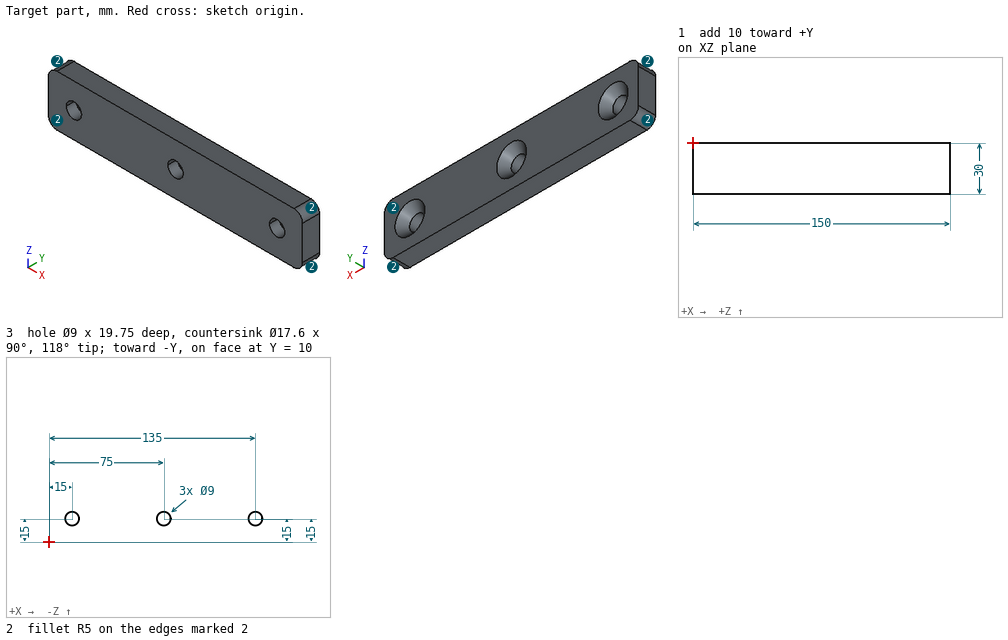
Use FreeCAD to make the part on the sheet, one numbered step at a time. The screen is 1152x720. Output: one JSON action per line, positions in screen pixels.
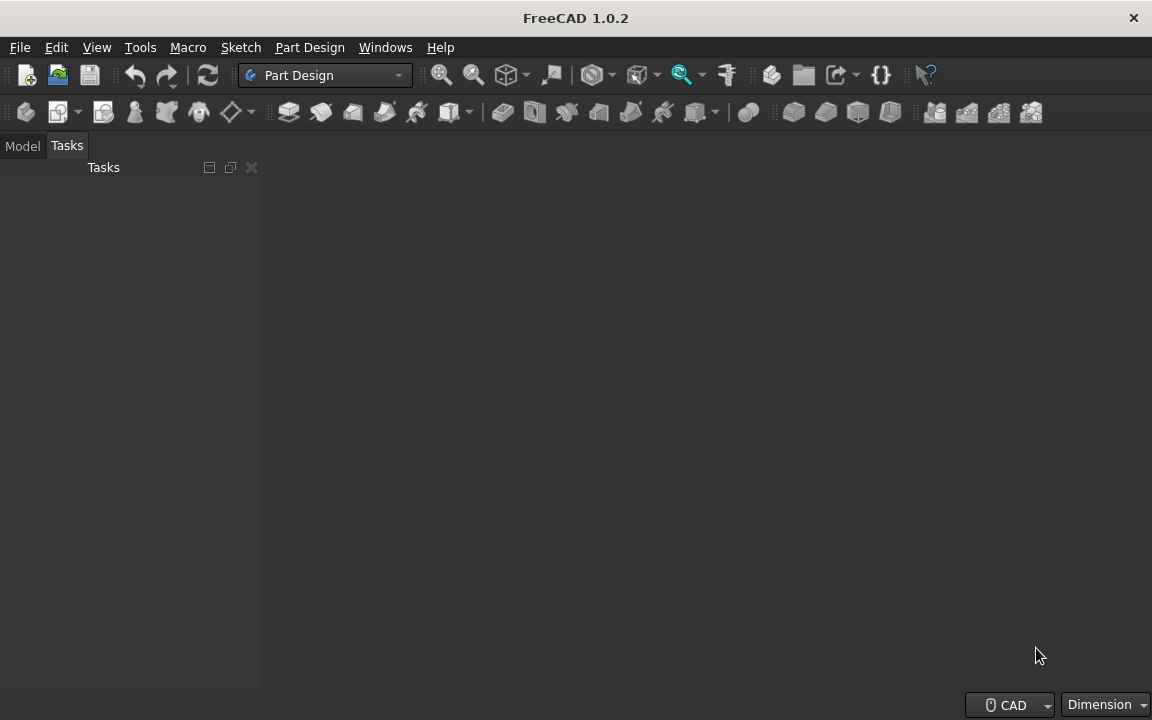
{"action": "left_click", "coordinate": [26, 76]}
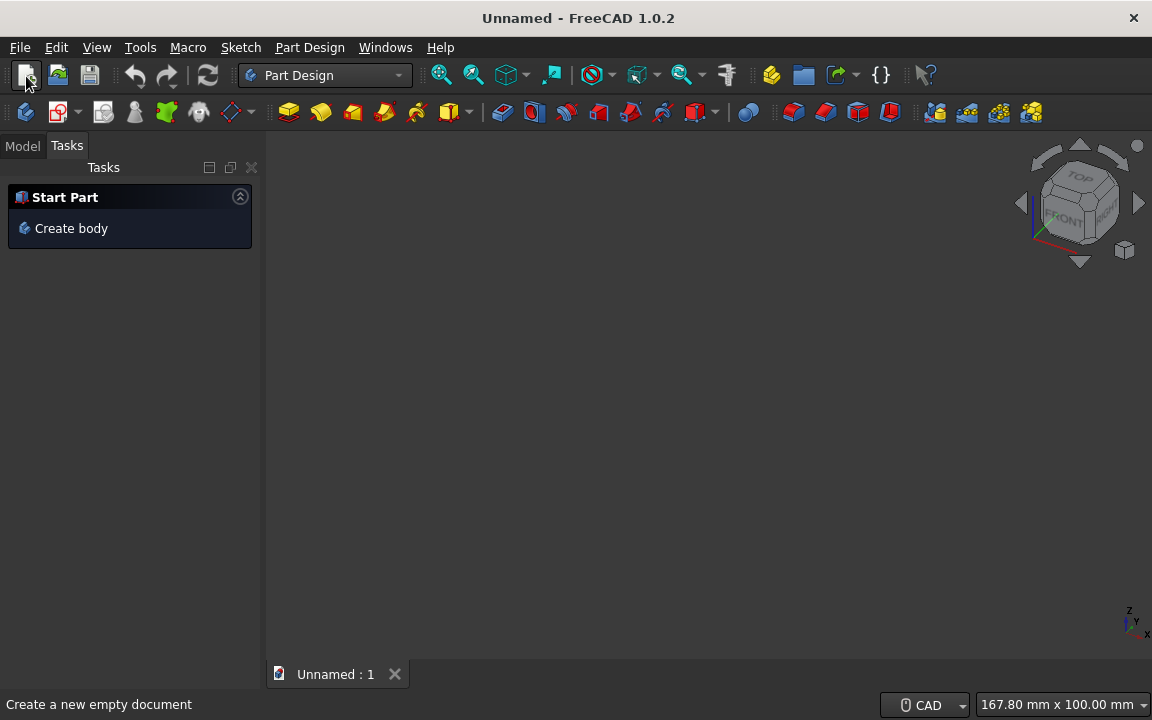
{"action": "left_click", "coordinate": [58, 112]}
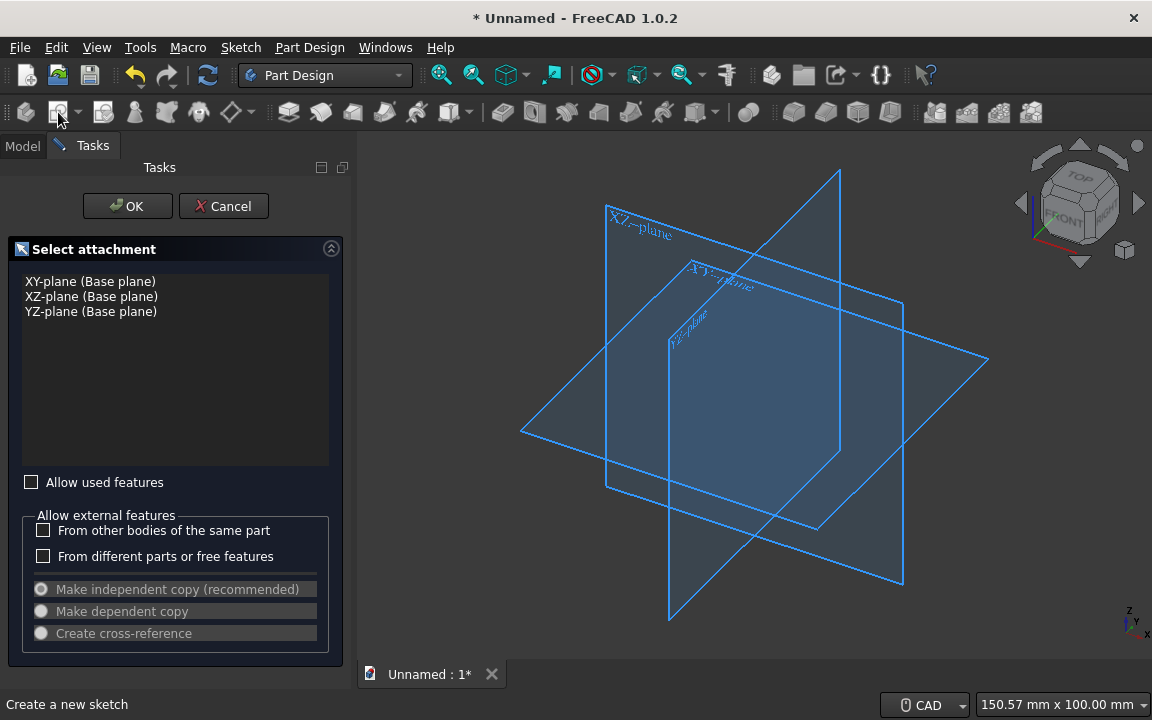
{"action": "left_click", "coordinate": [82, 296]}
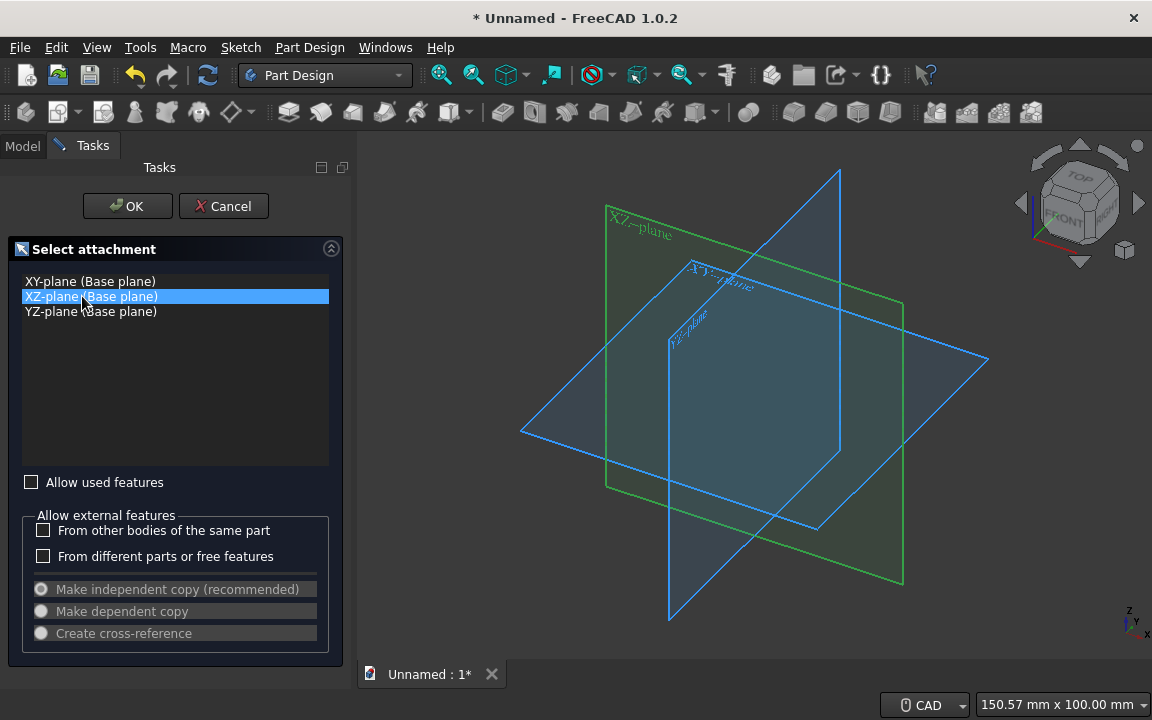
{"action": "left_click", "coordinate": [128, 206]}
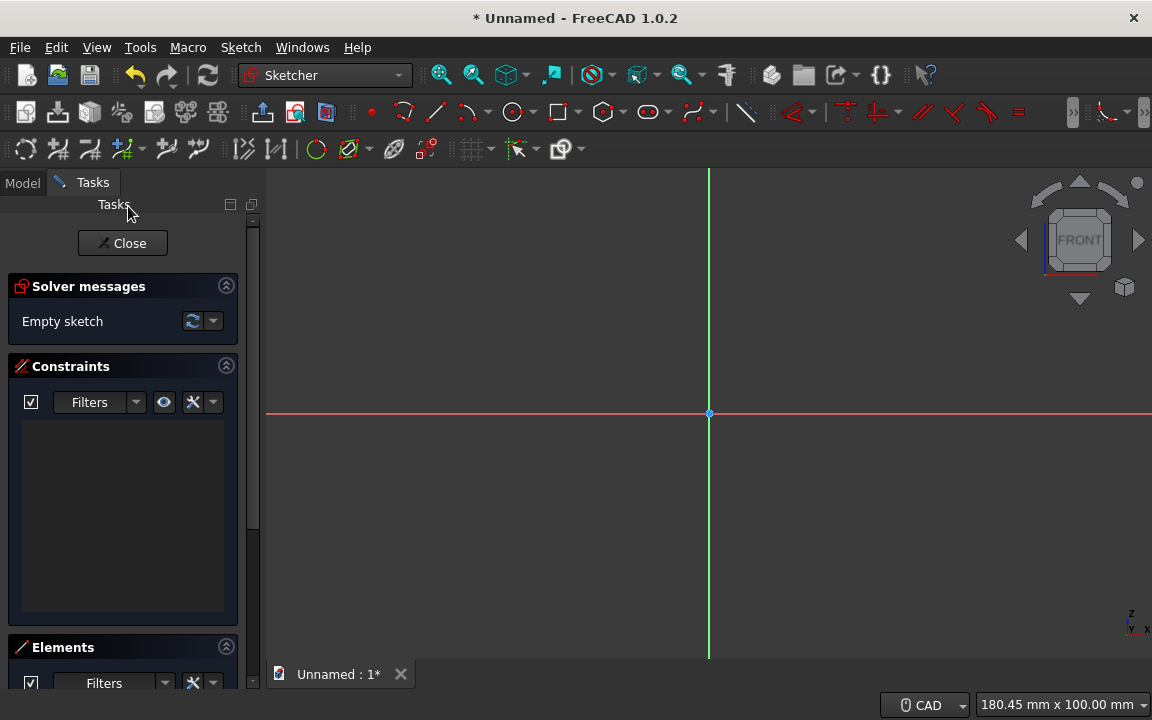
{"action": "scroll", "coordinate": [294, 324], "scroll_direction": "down", "scroll_amount": 3}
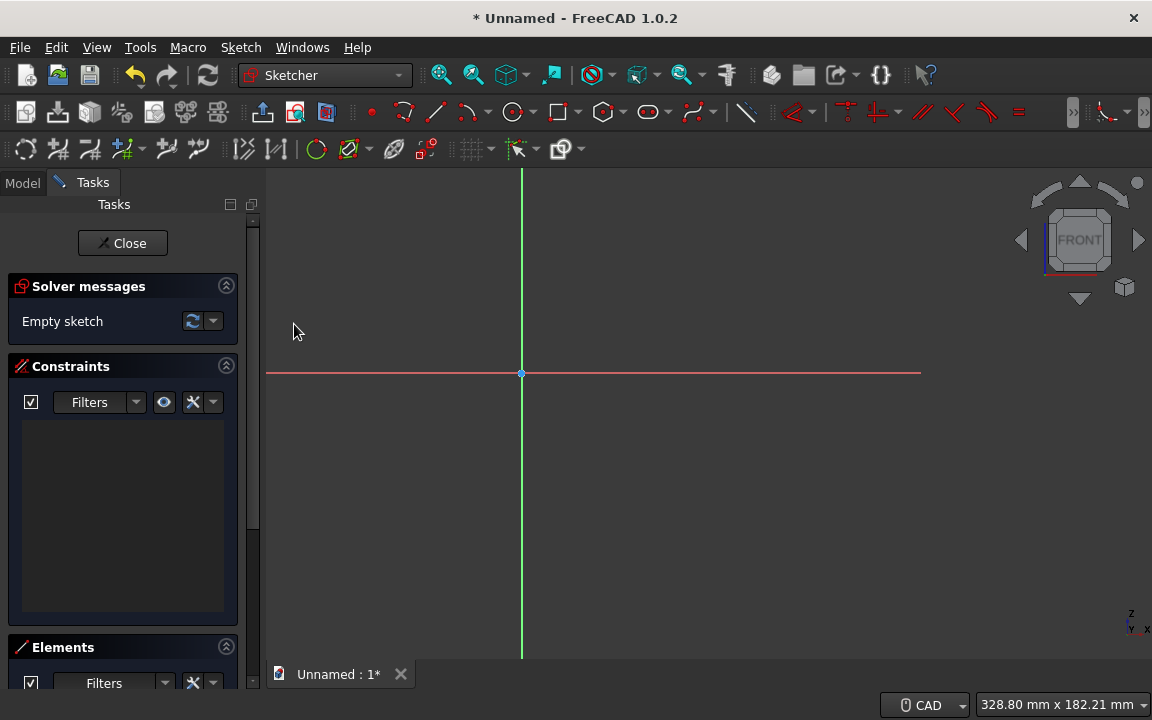
{"action": "left_click", "coordinate": [558, 112]}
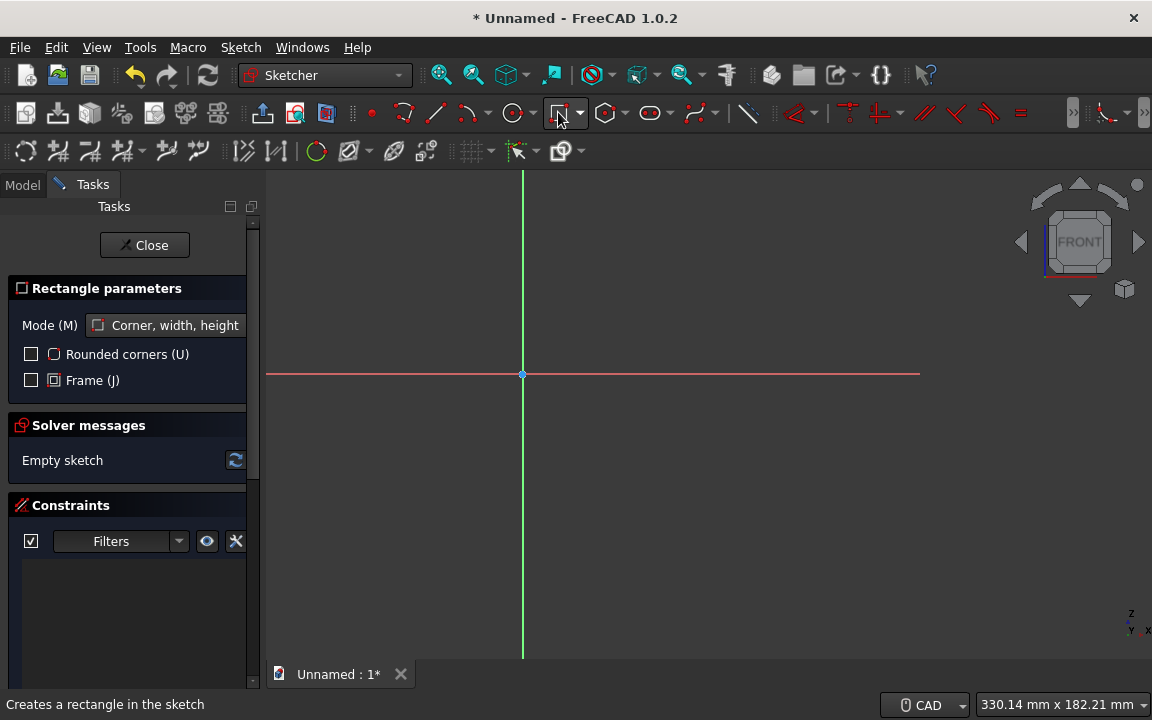
{"action": "left_click", "coordinate": [523, 374]}
{"action": "mouse_move", "coordinate": [925, 455]}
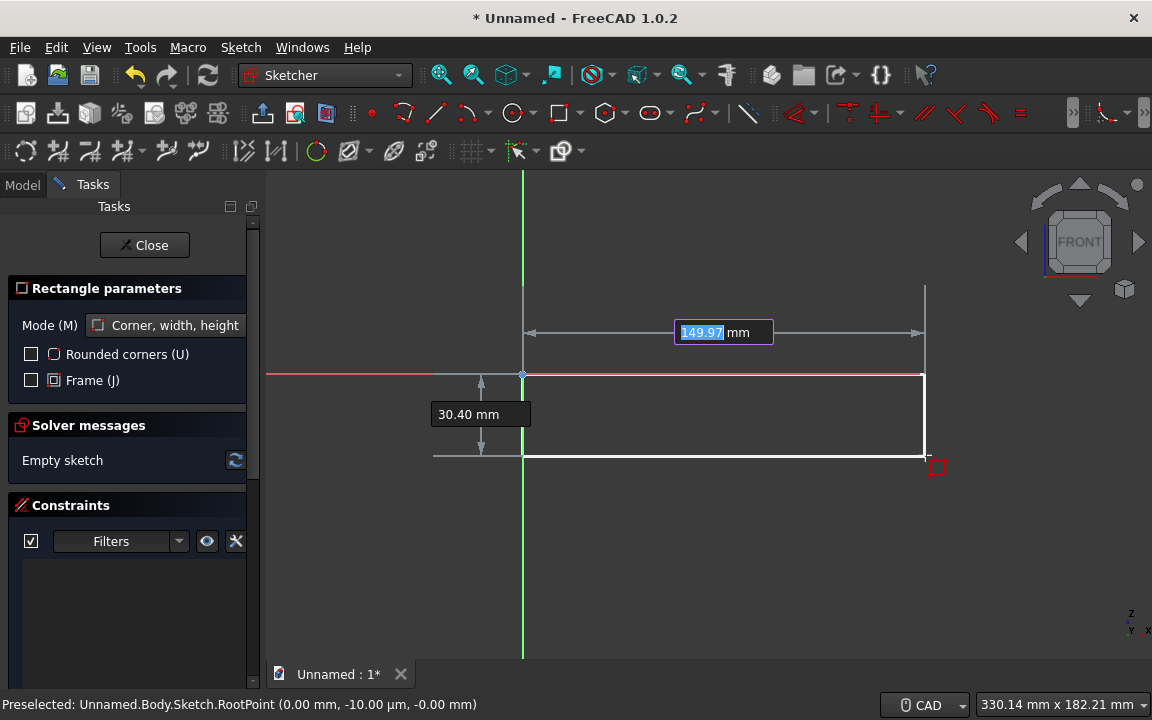
{"action": "type", "text": "150"}
{"action": "key", "text": "Tab"}
{"action": "type", "text": "30"}
{"action": "key", "text": "Return"}
{"action": "key", "text": "Escape"}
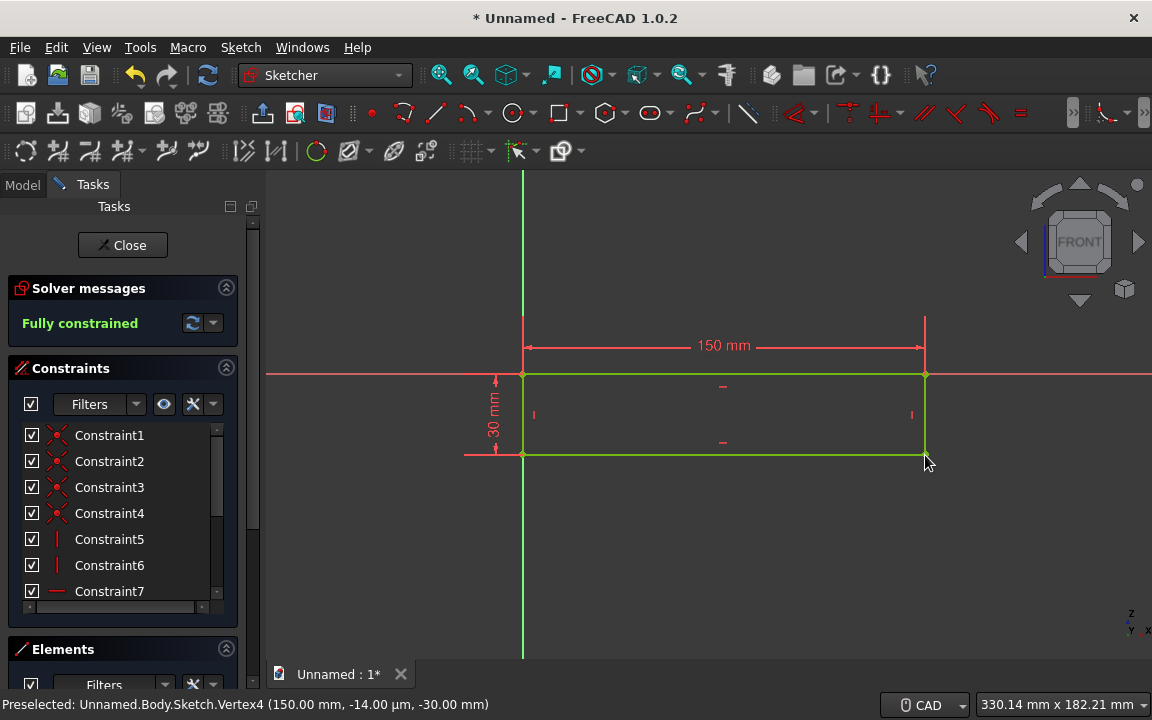
{"action": "left_click", "coordinate": [123, 245]}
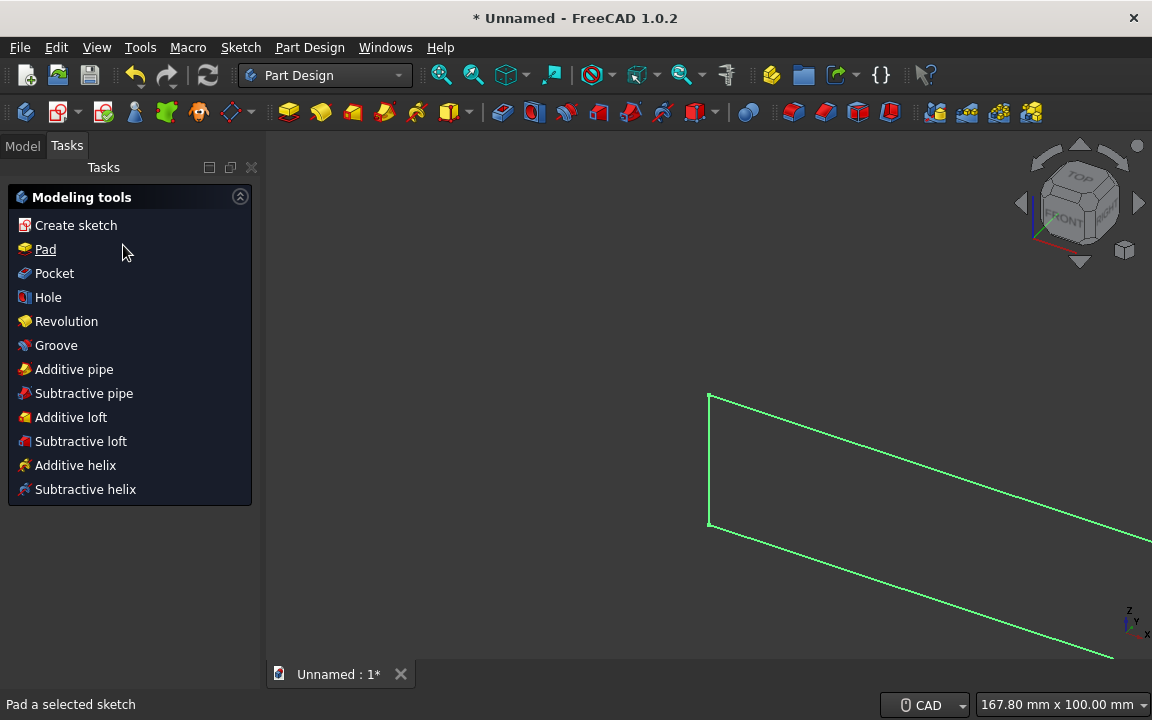
{"action": "left_click", "coordinate": [290, 112]}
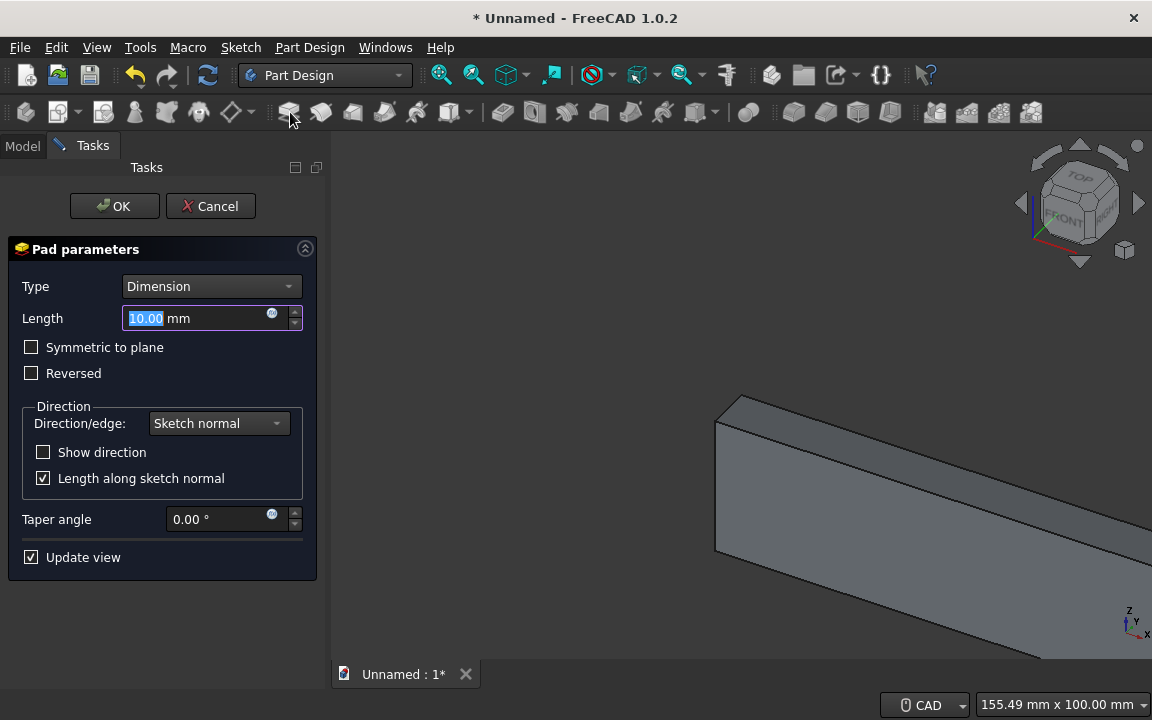
{"action": "type", "text": "10"}
{"action": "key", "text": "Tab"}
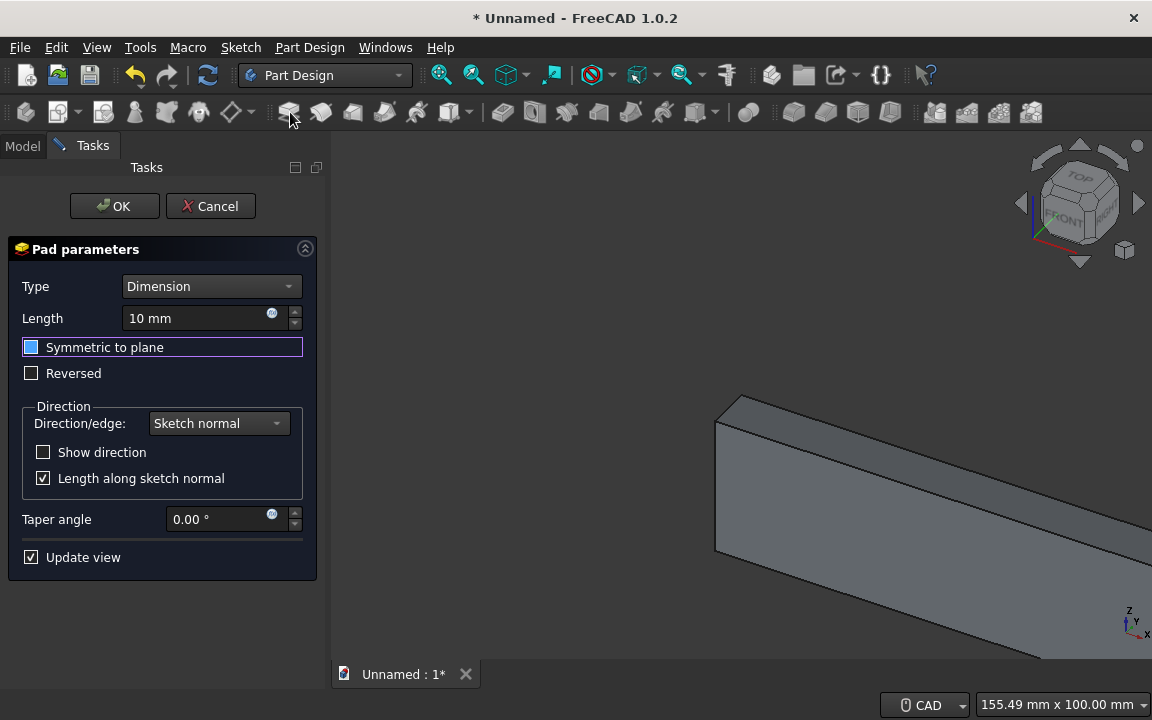
{"action": "left_click", "coordinate": [30, 373]}